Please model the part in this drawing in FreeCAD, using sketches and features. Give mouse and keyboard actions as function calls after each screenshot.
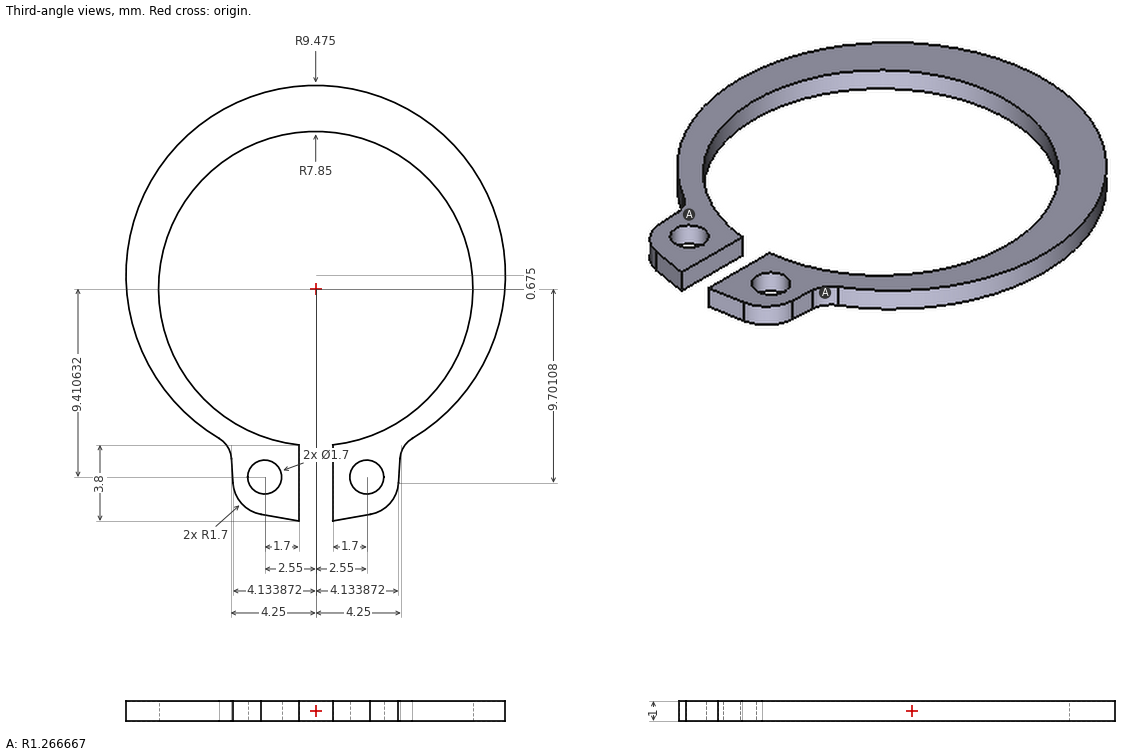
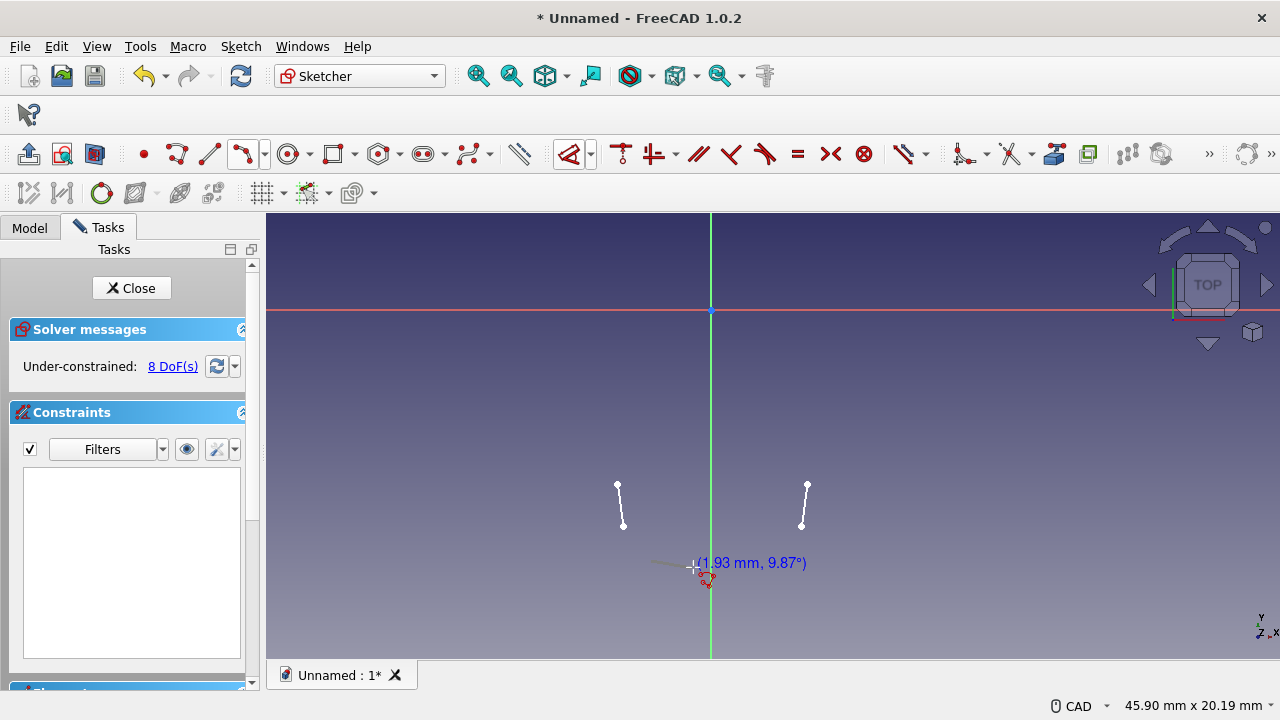
click(693, 567)
click(693, 483)
right_click(693, 483)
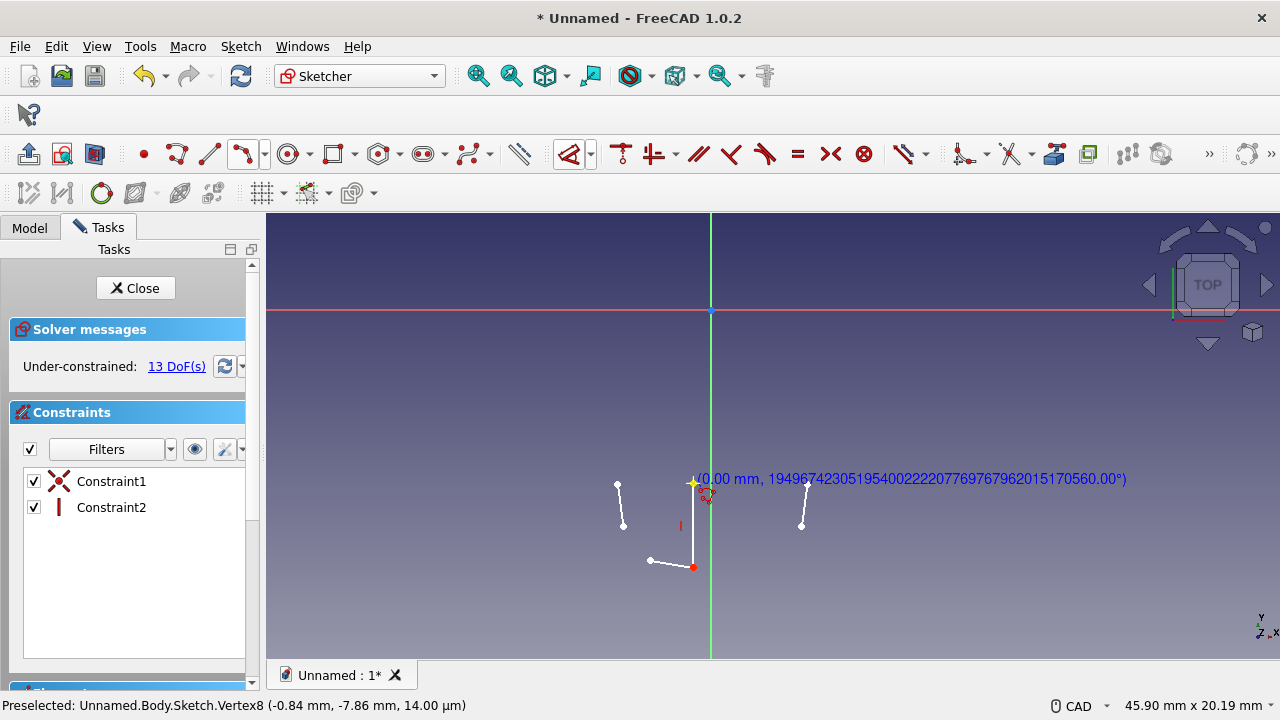
click(730, 483)
click(730, 567)
click(772, 559)
right_click(772, 559)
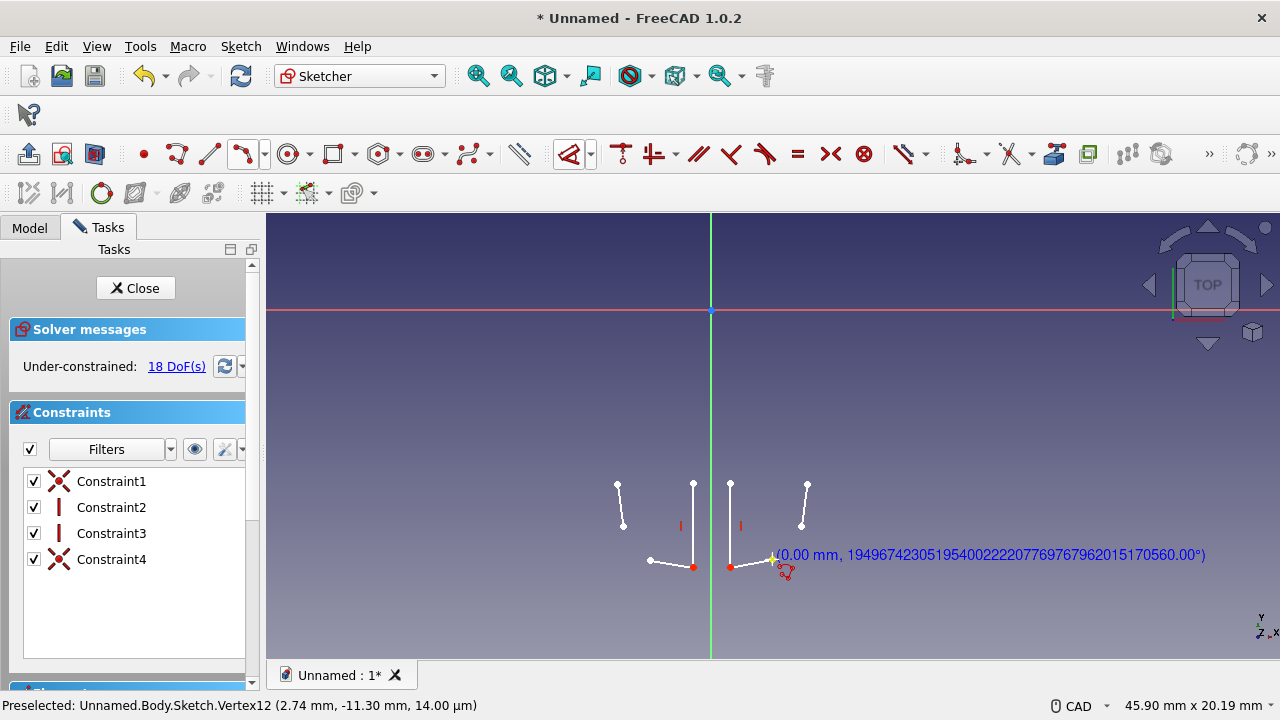
click(242, 154)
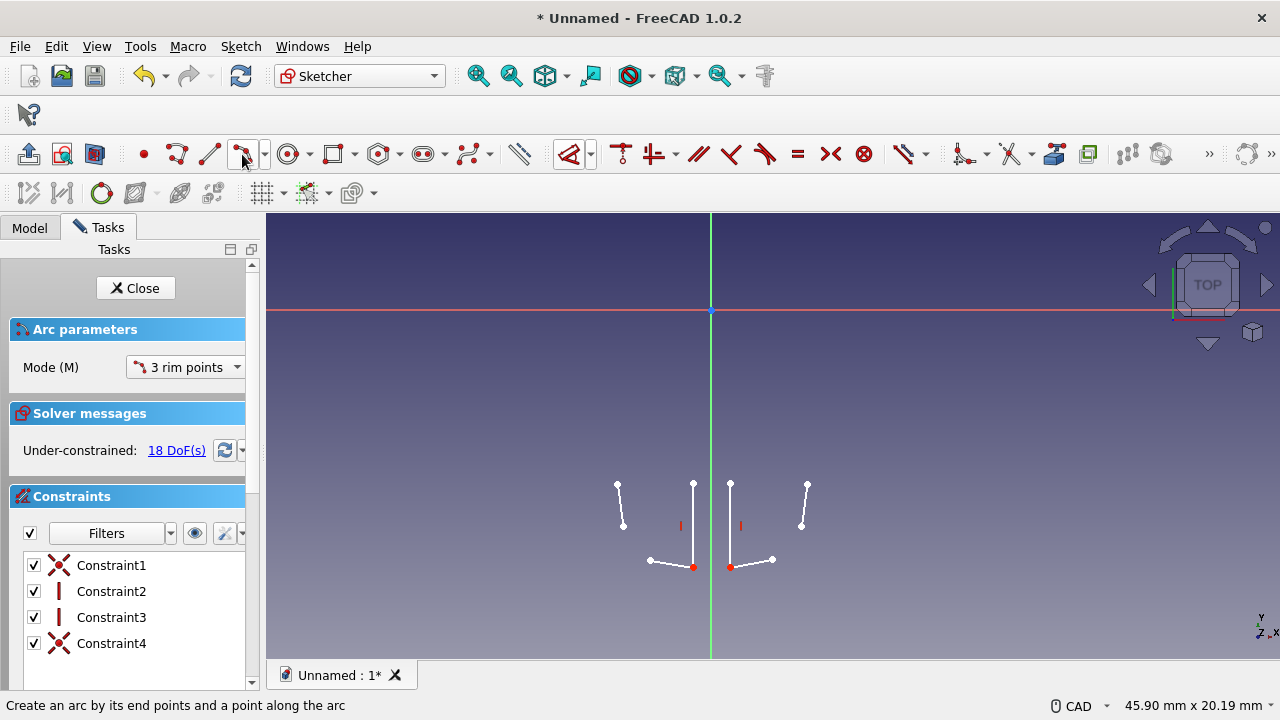
click(807, 484)
click(618, 484)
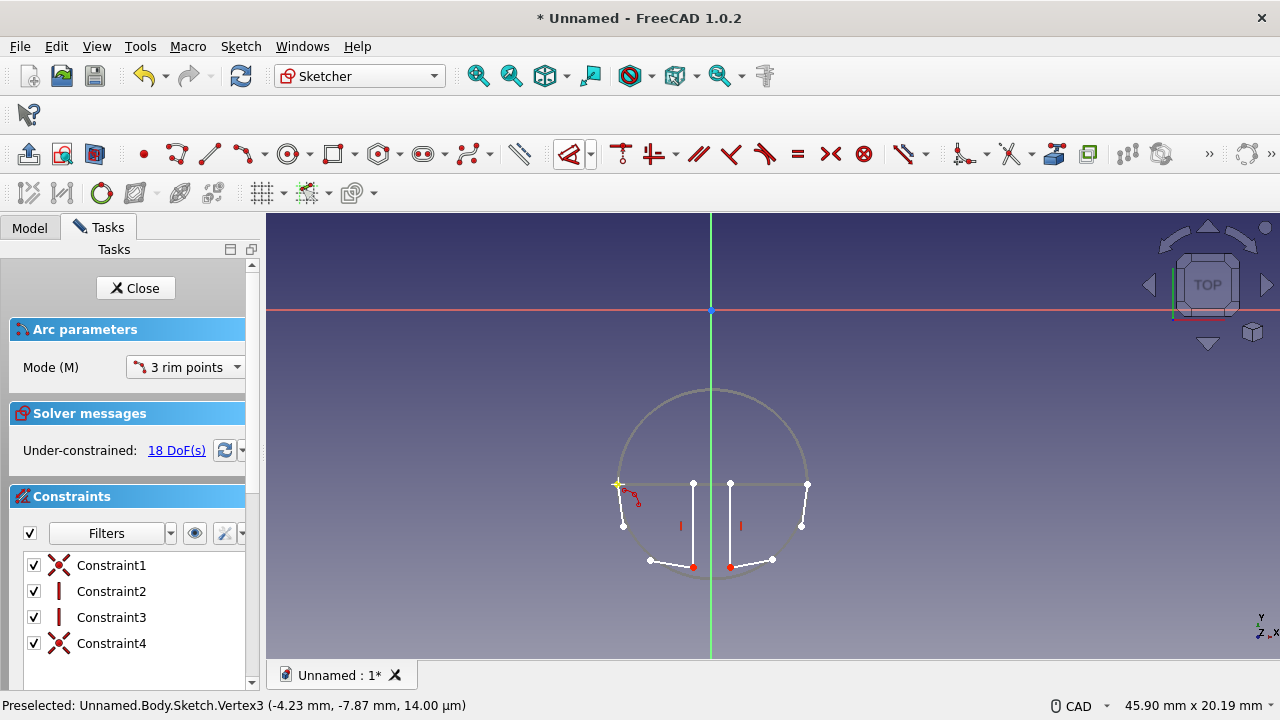
scroll(696, 569, down, 3)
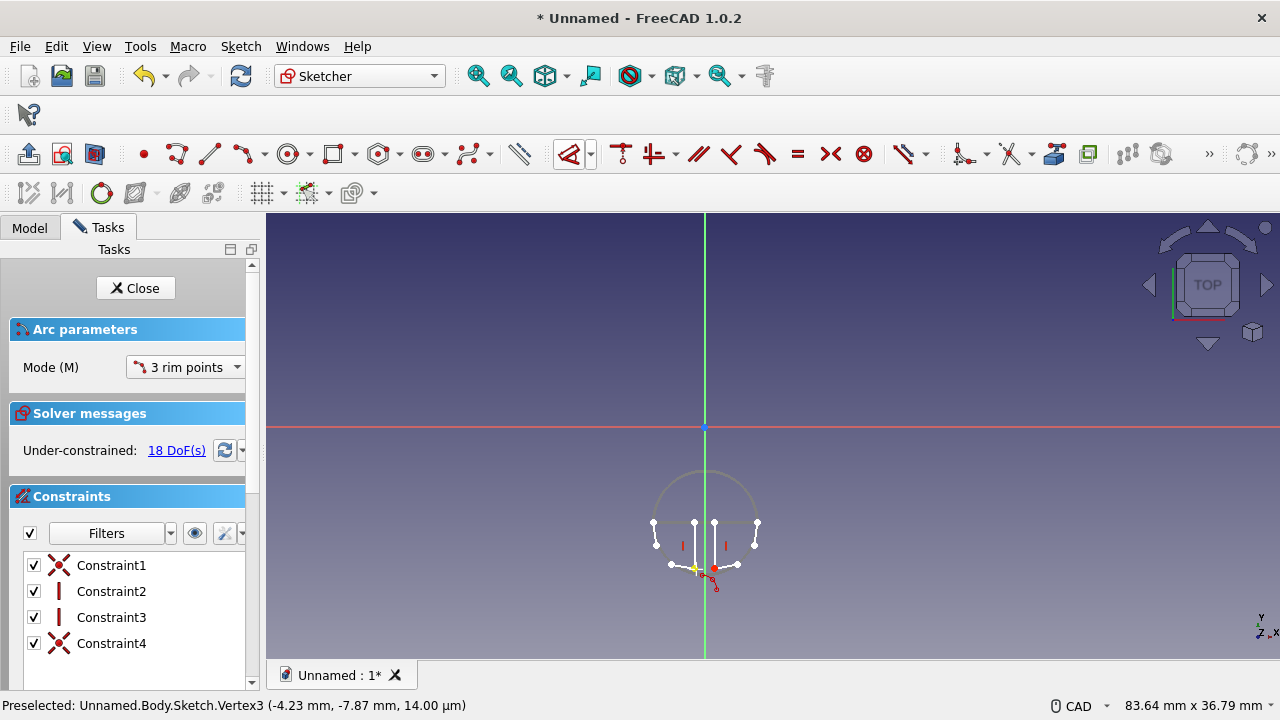
click(763, 320)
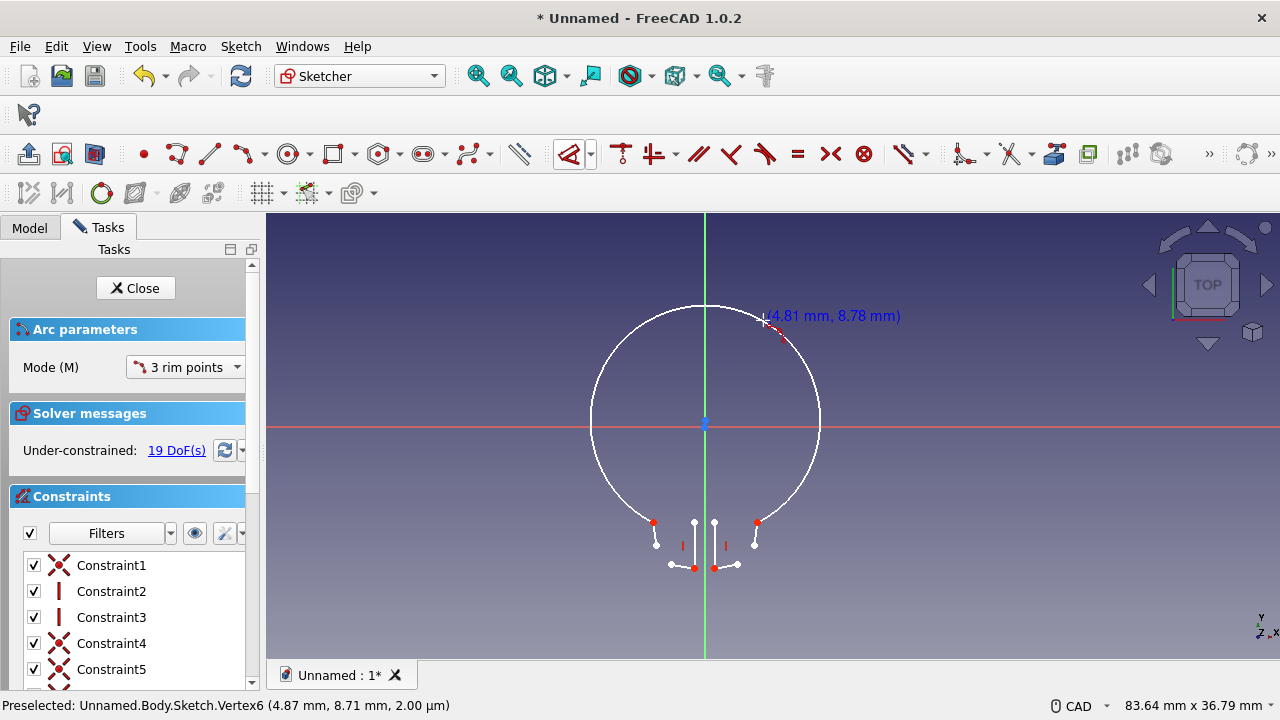
scroll(655, 545, up, 2)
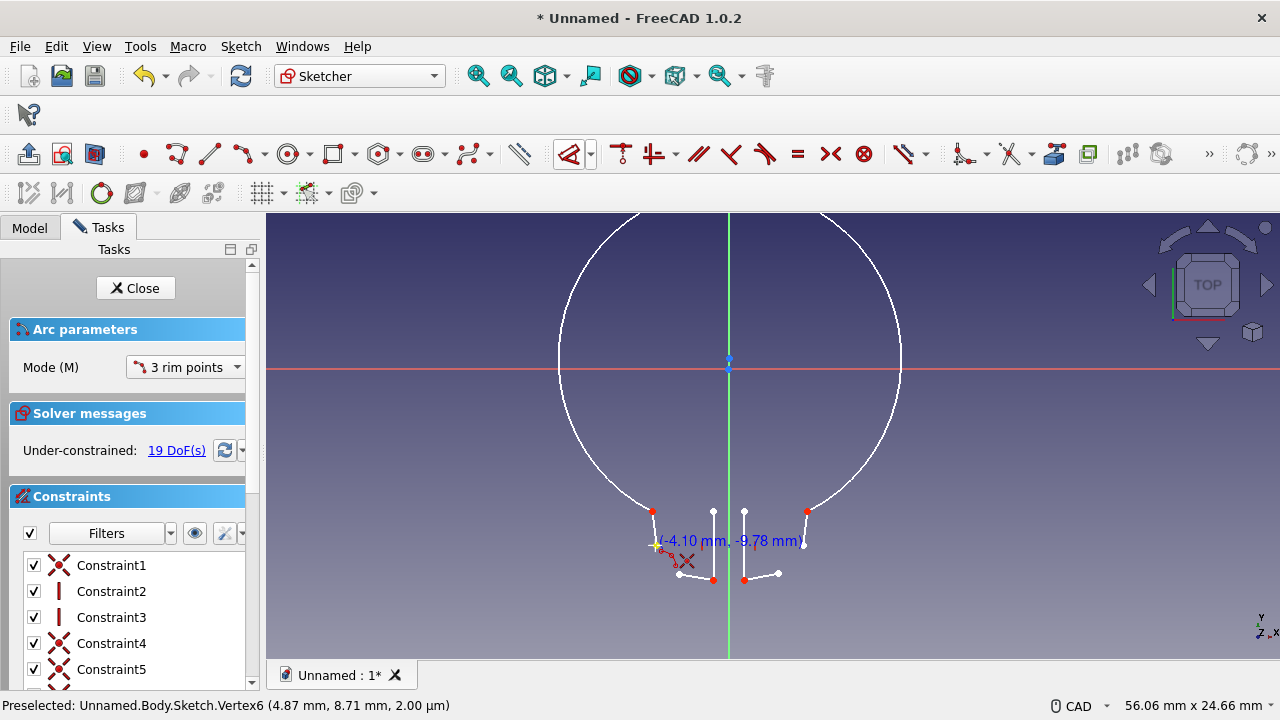
click(657, 546)
click(679, 574)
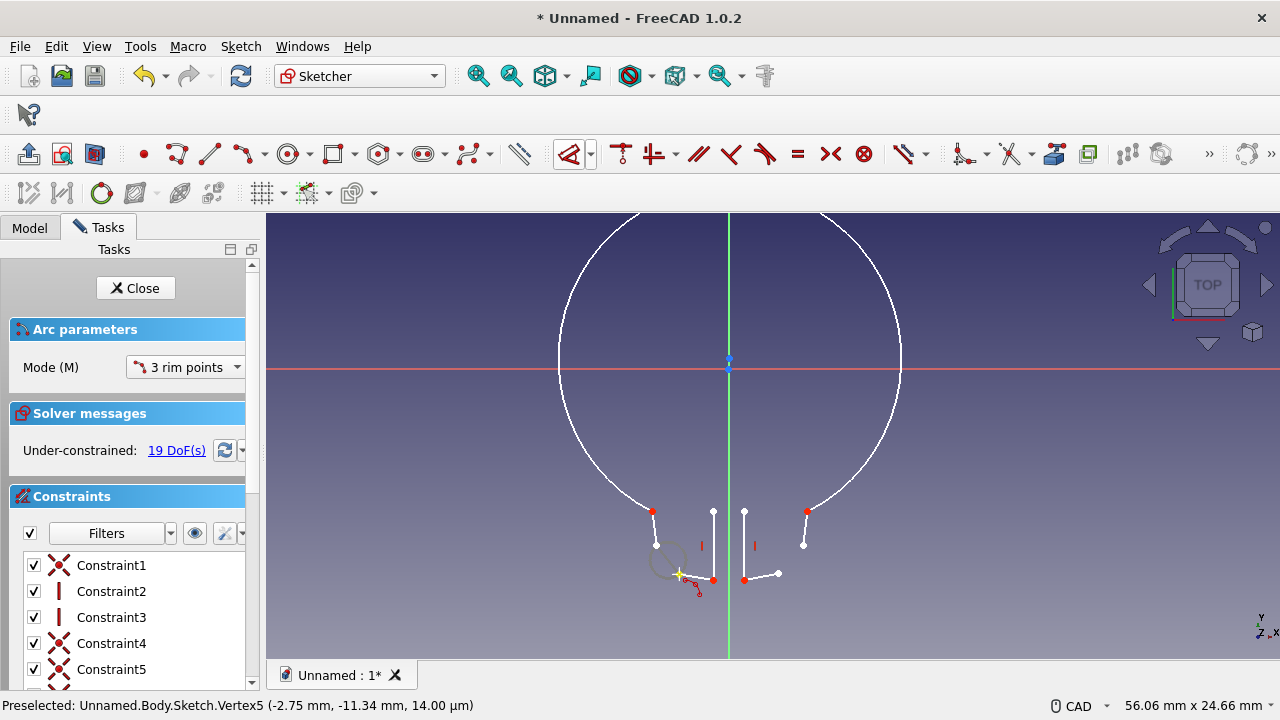
scroll(662, 563, up, 5)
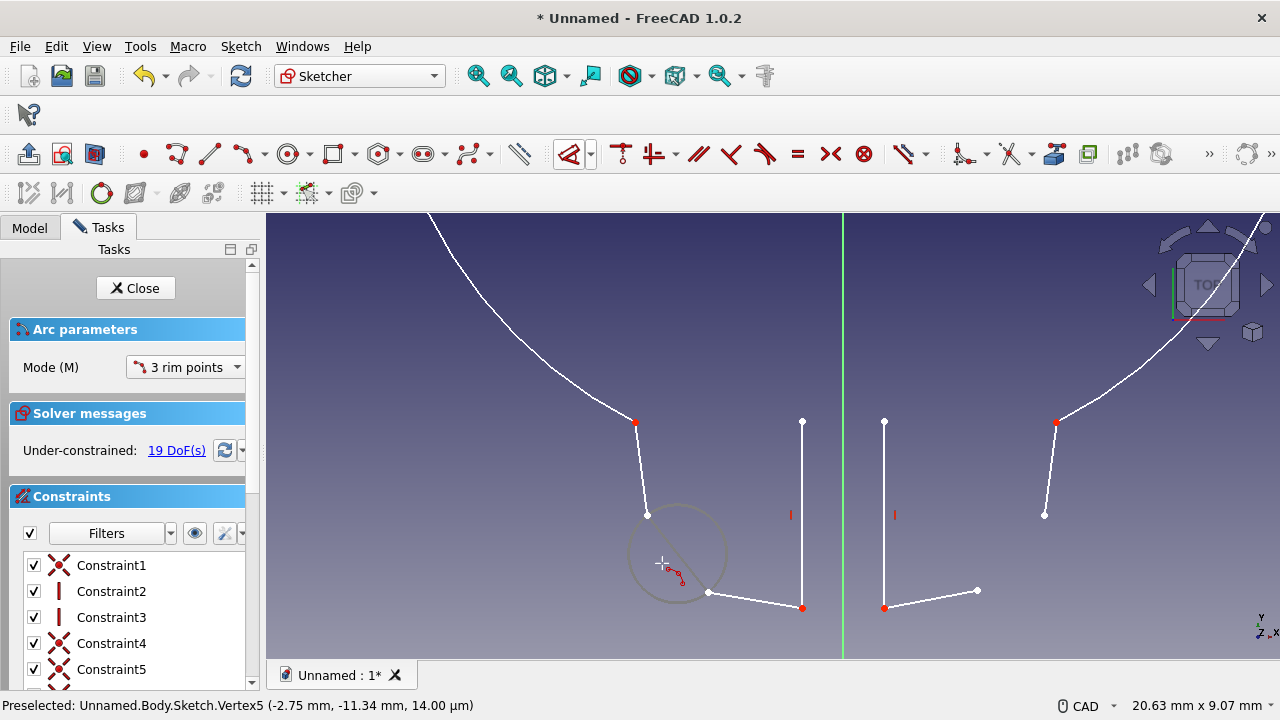
click(661, 562)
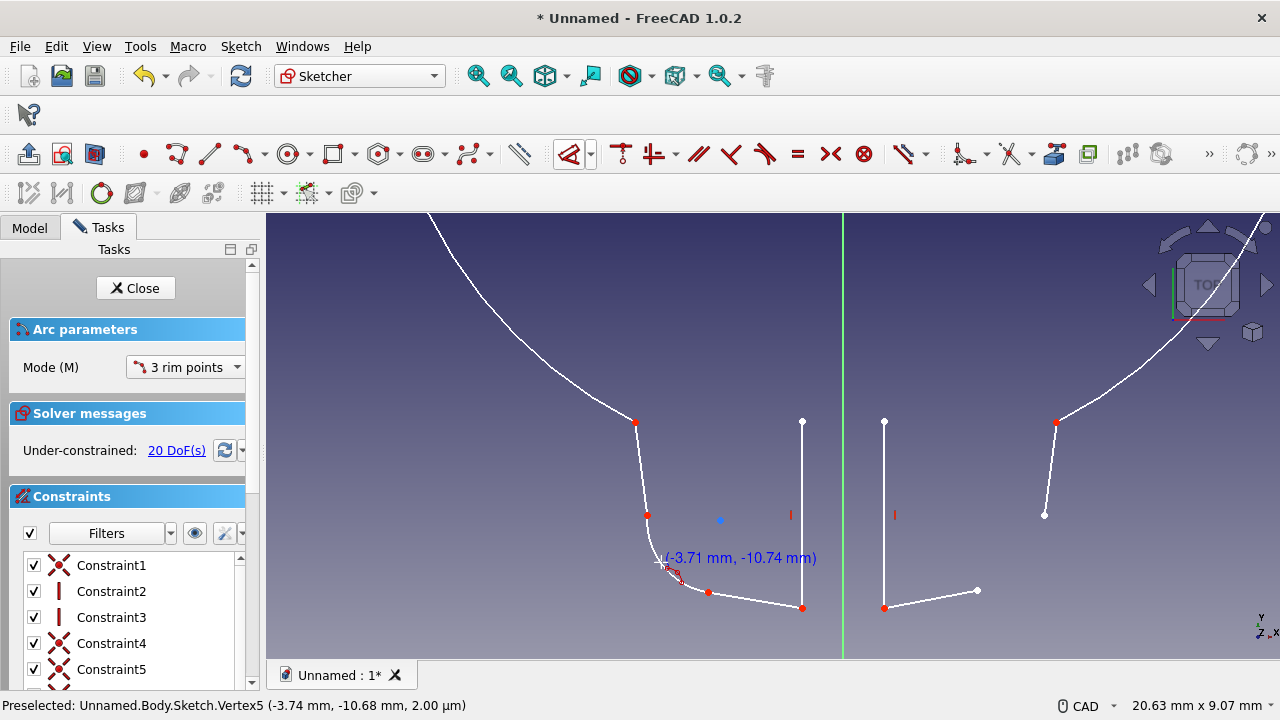
click(802, 421)
click(884, 421)